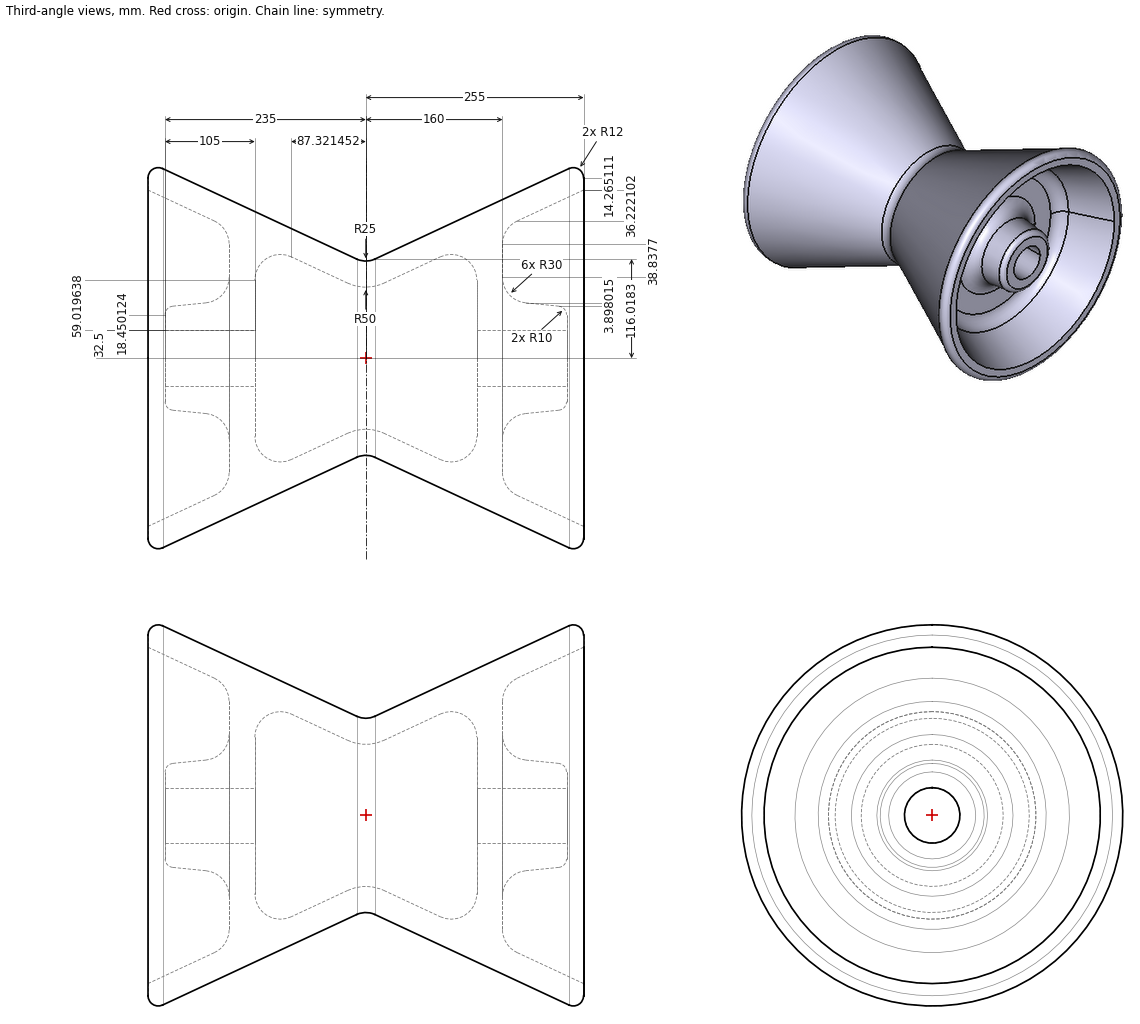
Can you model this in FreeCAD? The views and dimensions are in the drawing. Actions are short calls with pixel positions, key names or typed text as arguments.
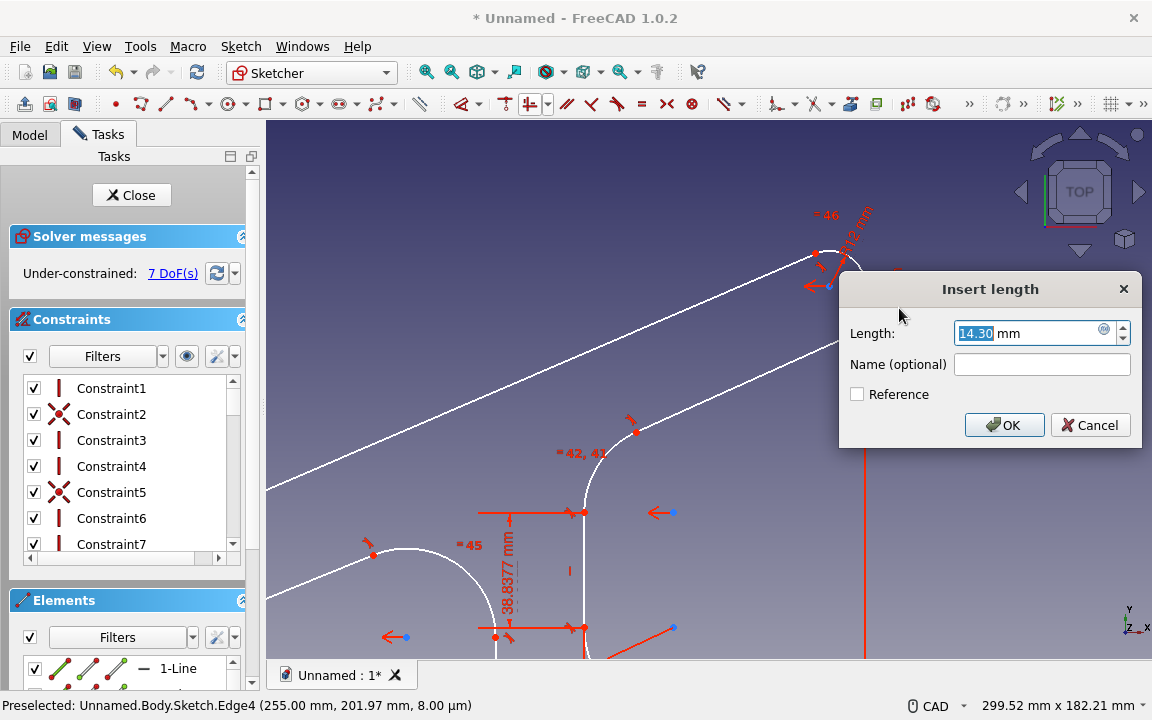
text(14.265111)
key(Return)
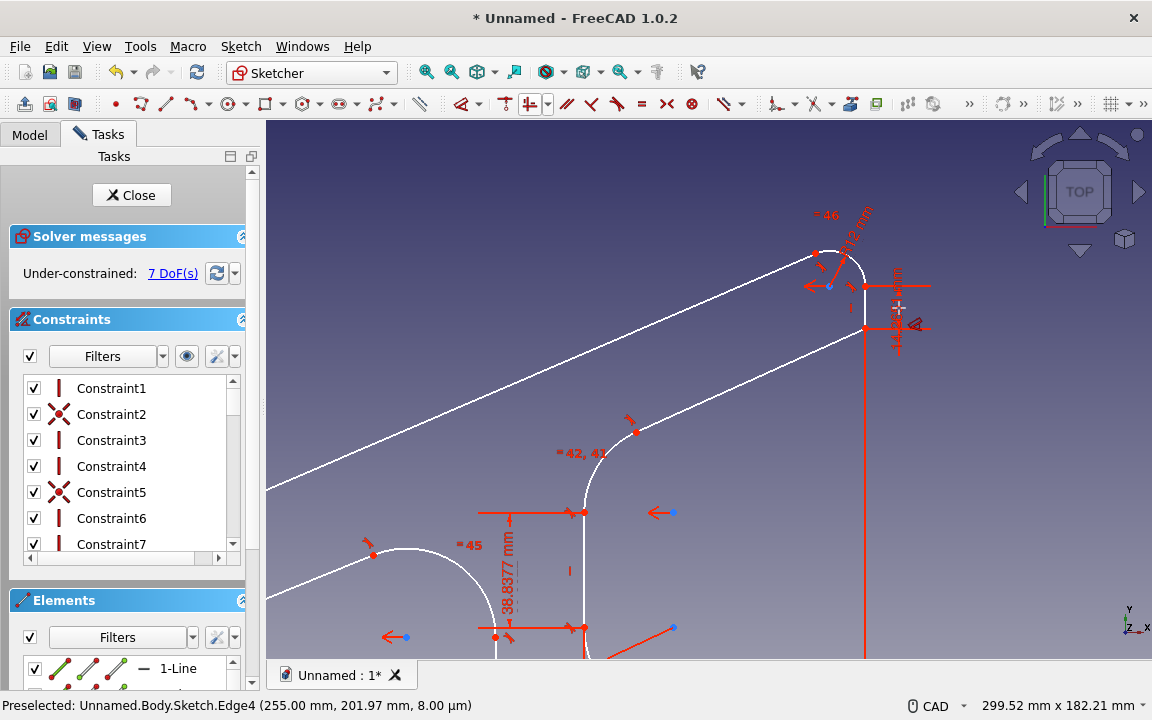
scroll(869, 308, down, 6)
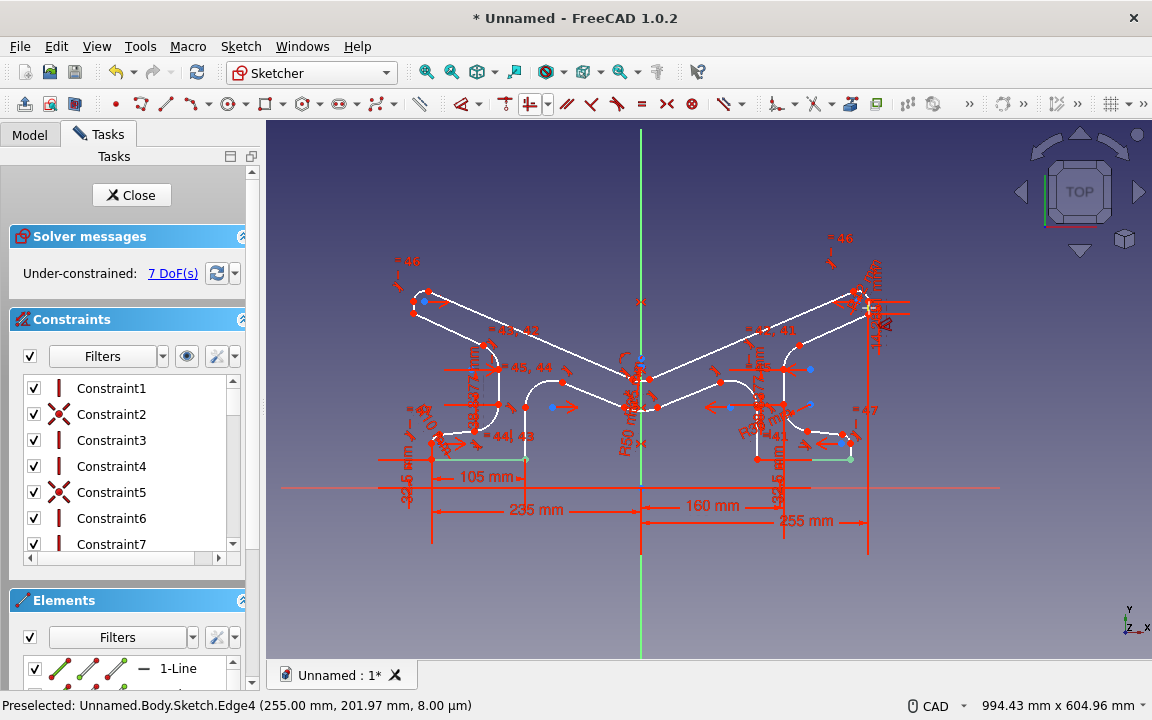
scroll(414, 305, up, 7)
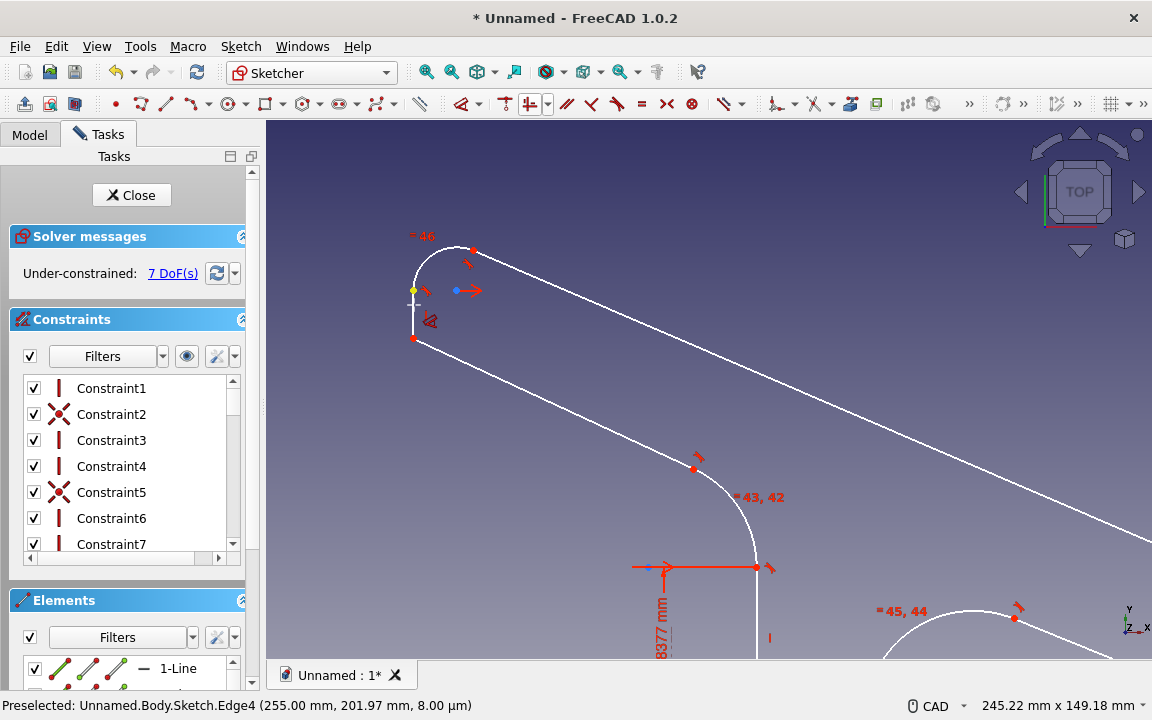
click(413, 305)
click(379, 315)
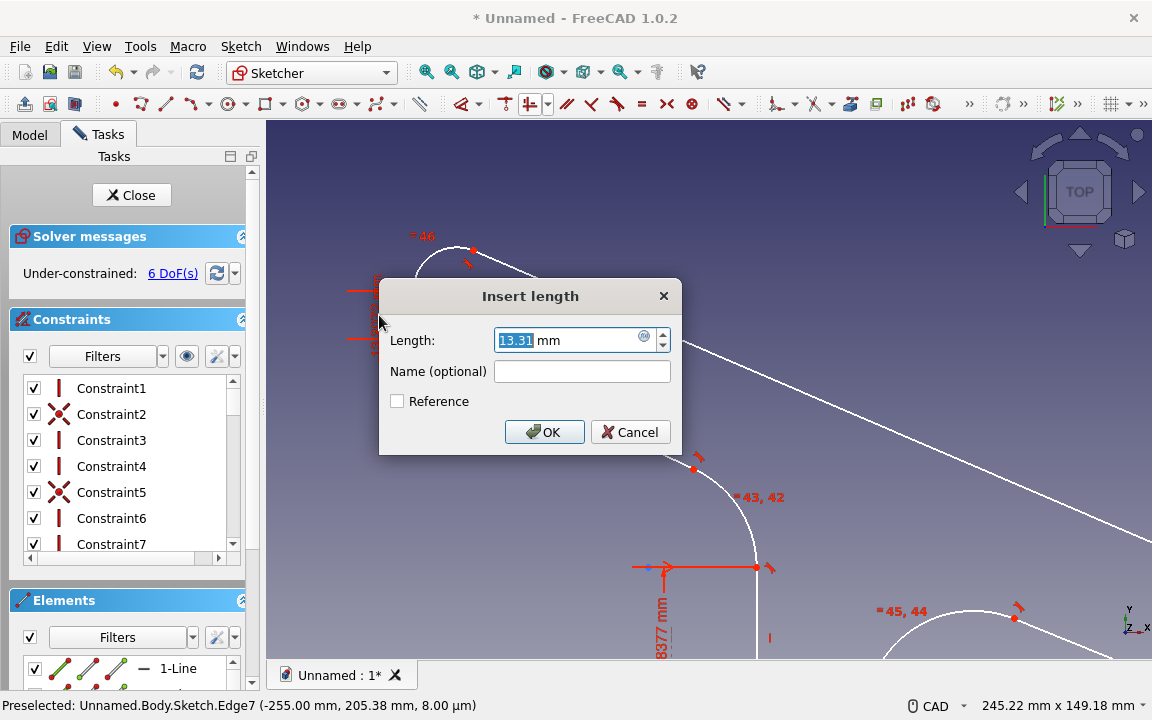
text(14.265111)
key(Return)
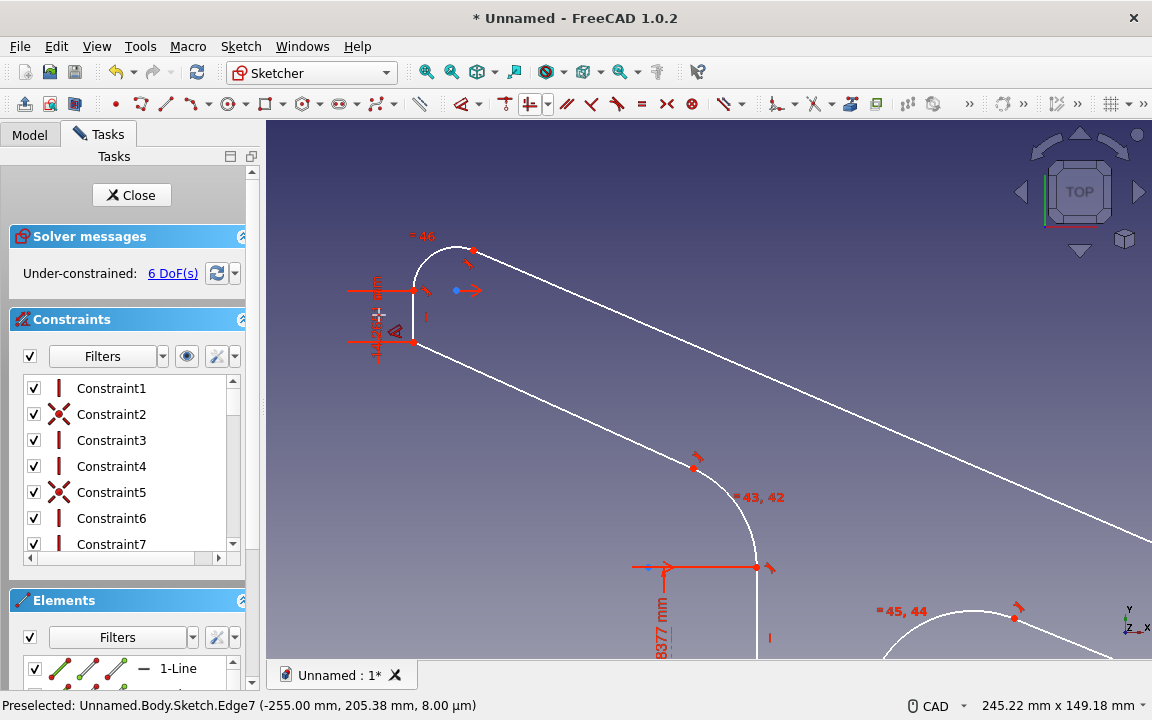
scroll(413, 305, down, 7)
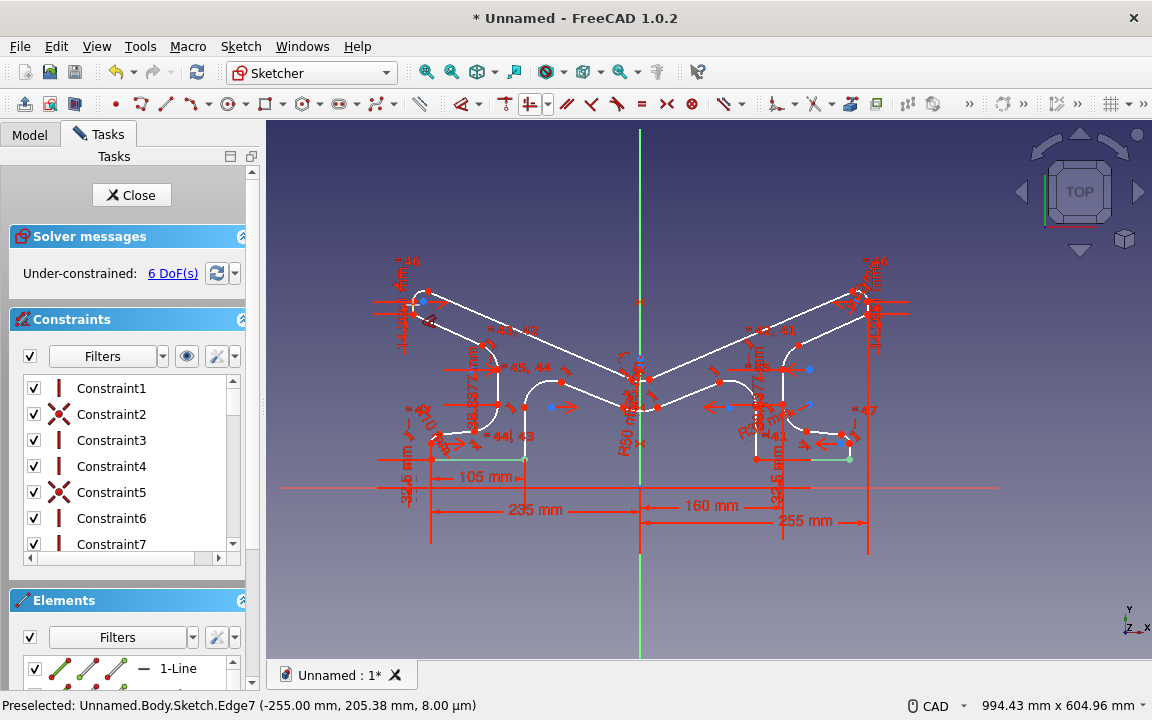
scroll(431, 449, up, 6)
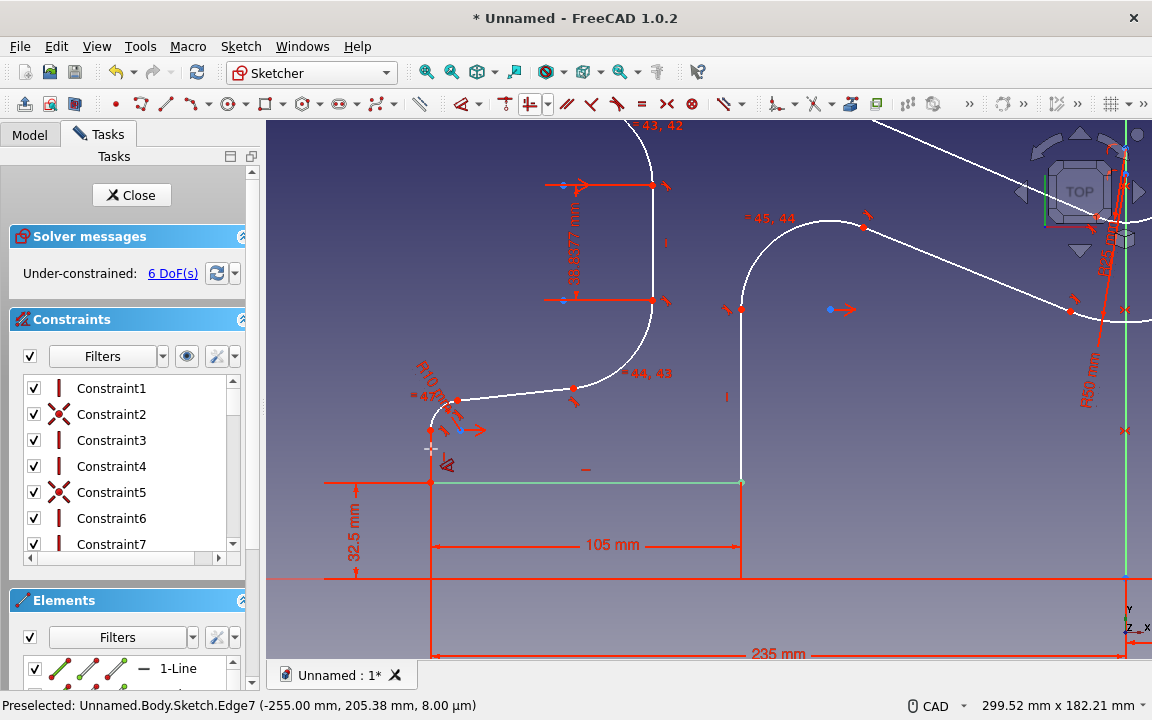
click(431, 446)
click(397, 456)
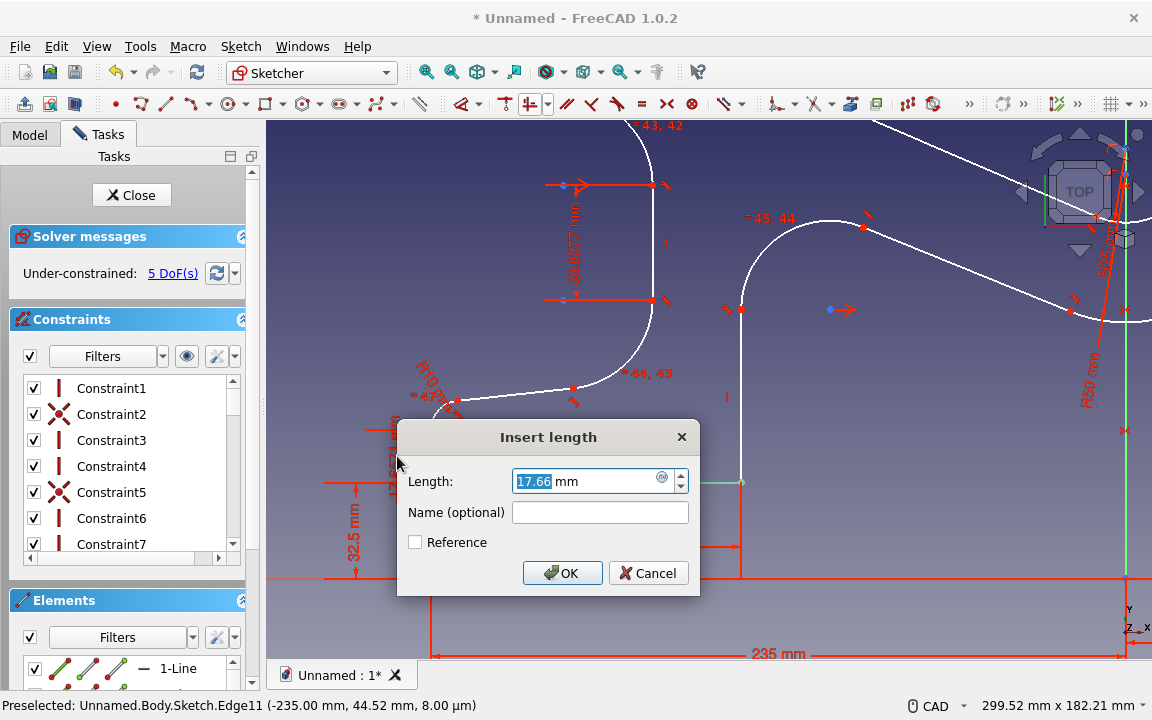
text(18.450124)
key(Return)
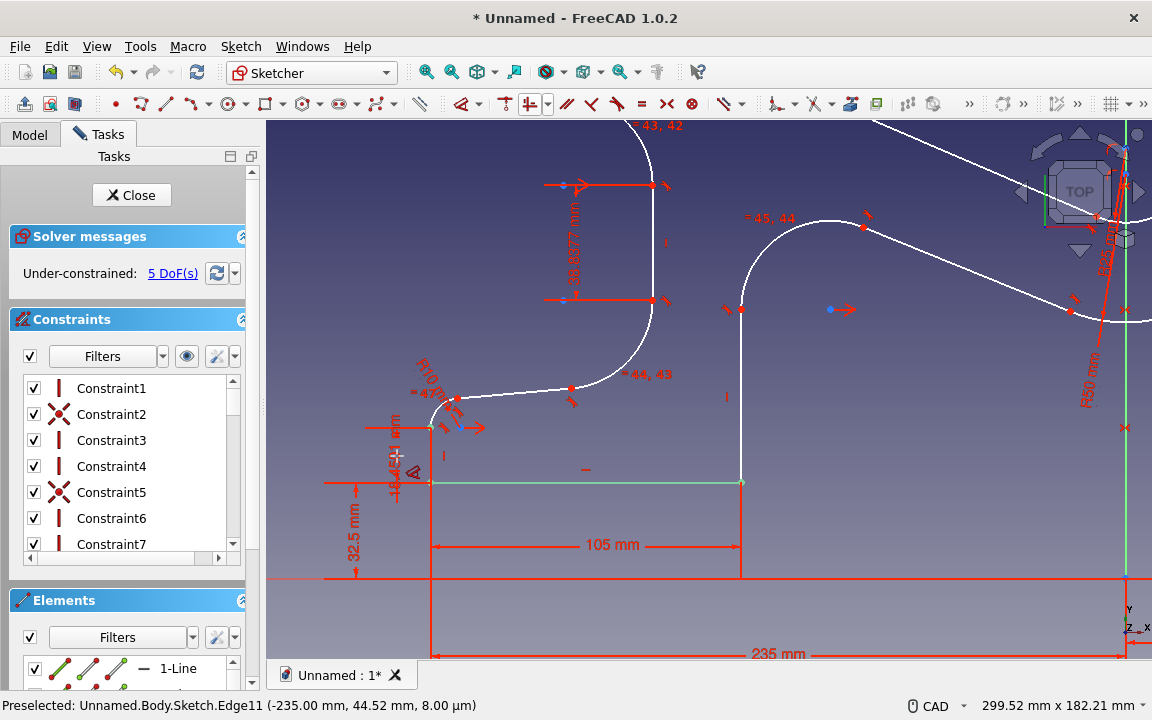
click(741, 431)
click(707, 396)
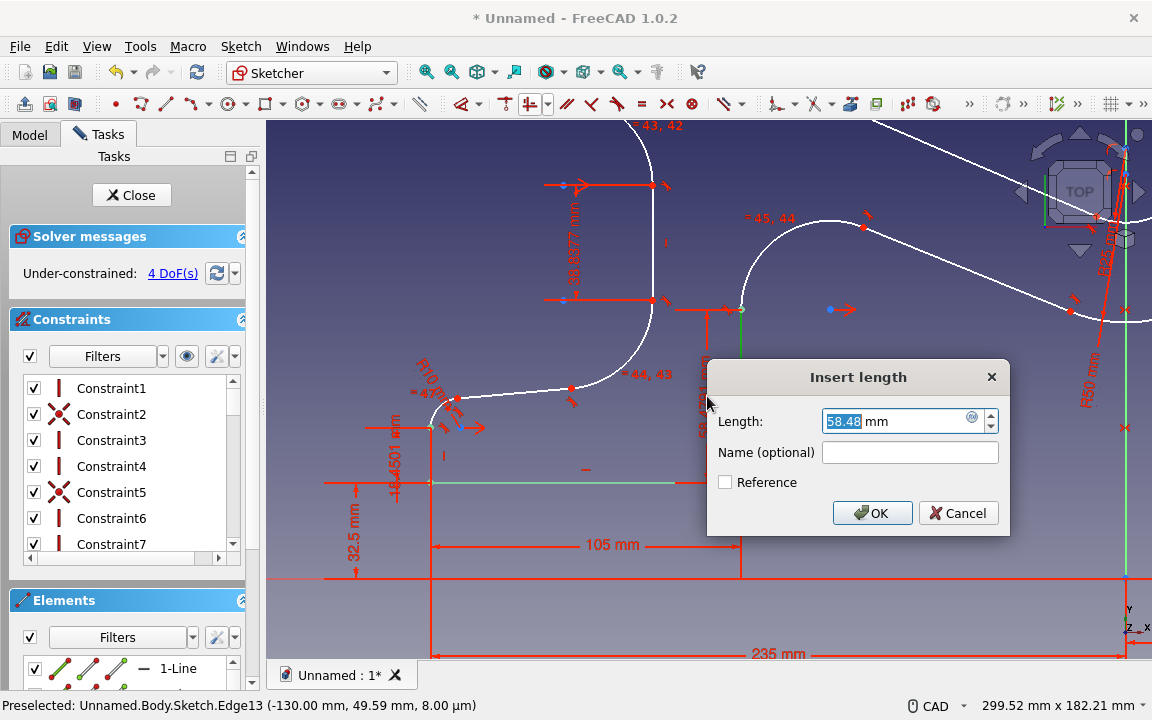
text(59.019638)
key(Return)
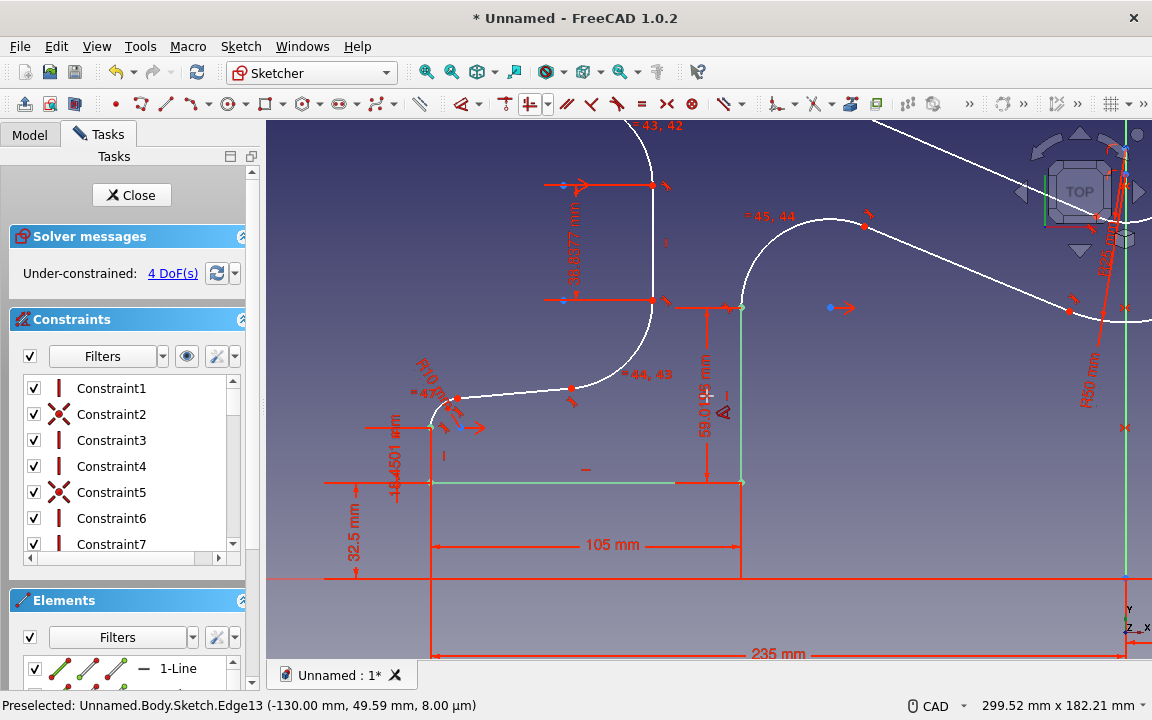
scroll(431, 449, down, 6)